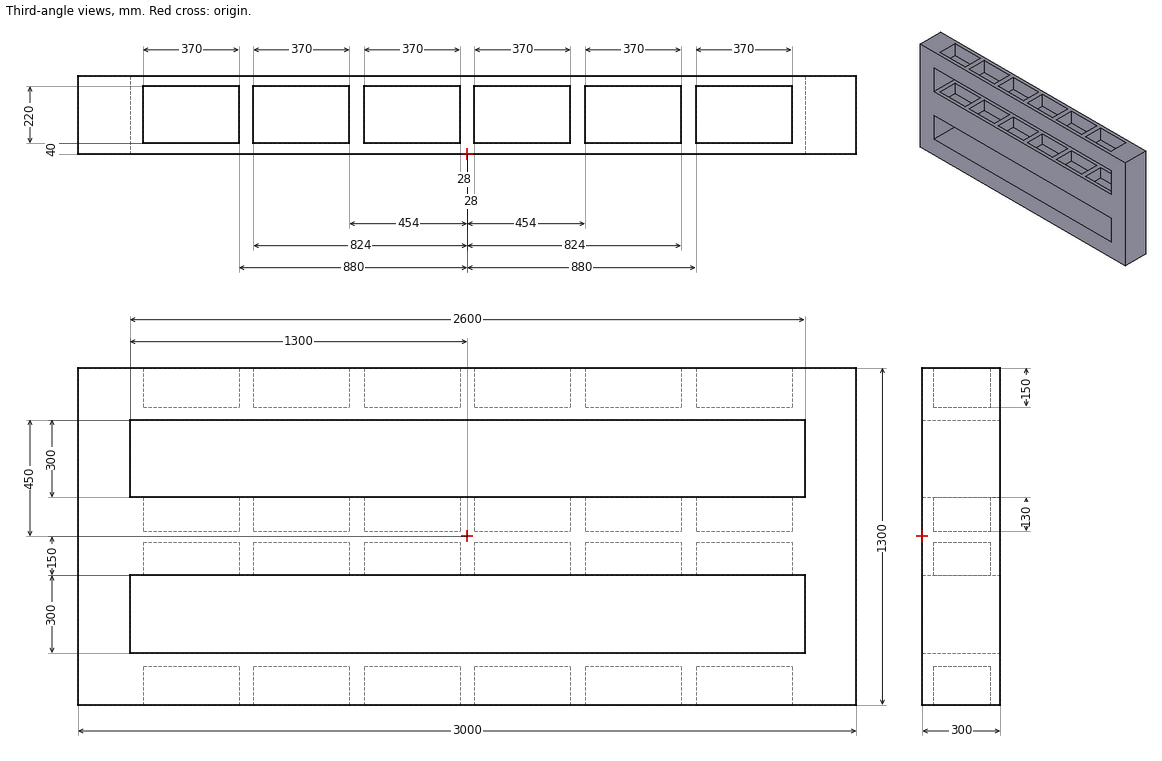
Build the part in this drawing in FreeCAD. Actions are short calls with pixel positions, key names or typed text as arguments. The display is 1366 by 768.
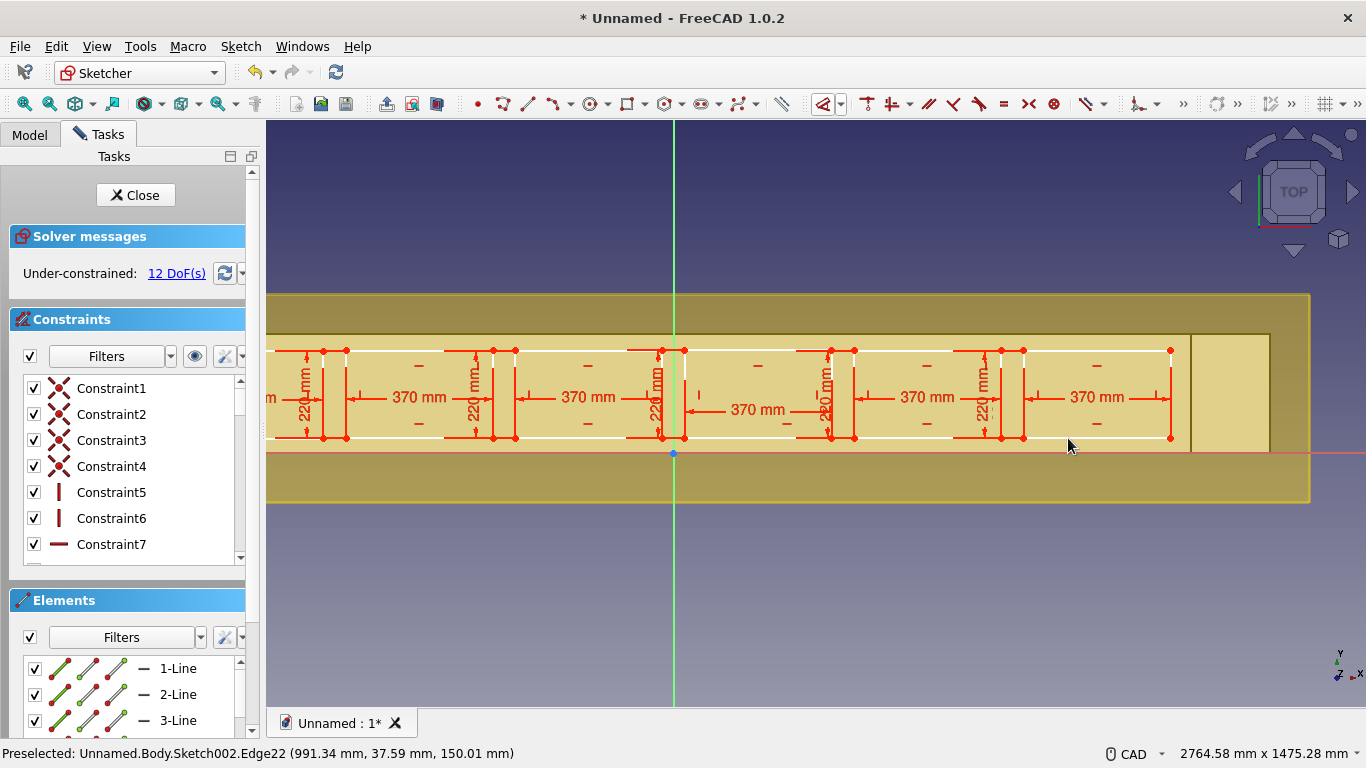
scroll(898, 438, down, 2)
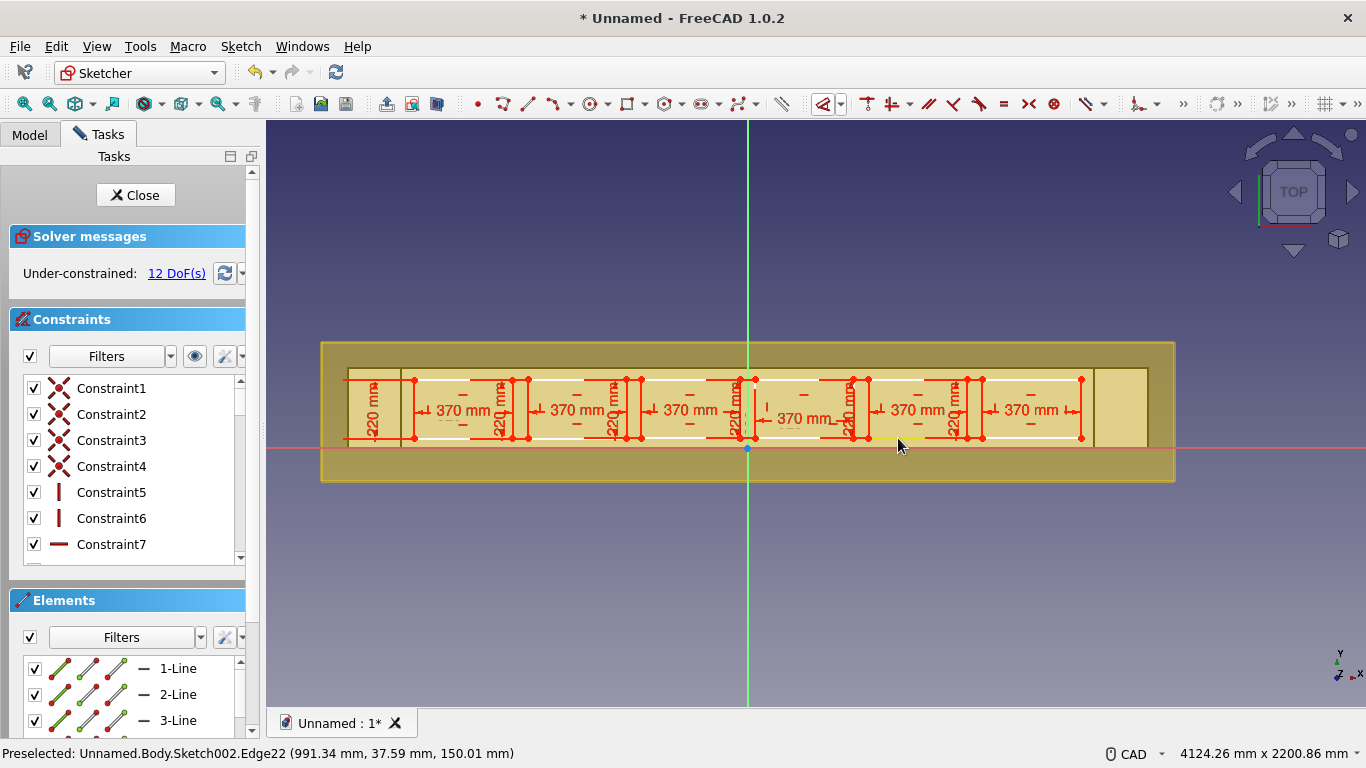
scroll(414, 439, up, 7)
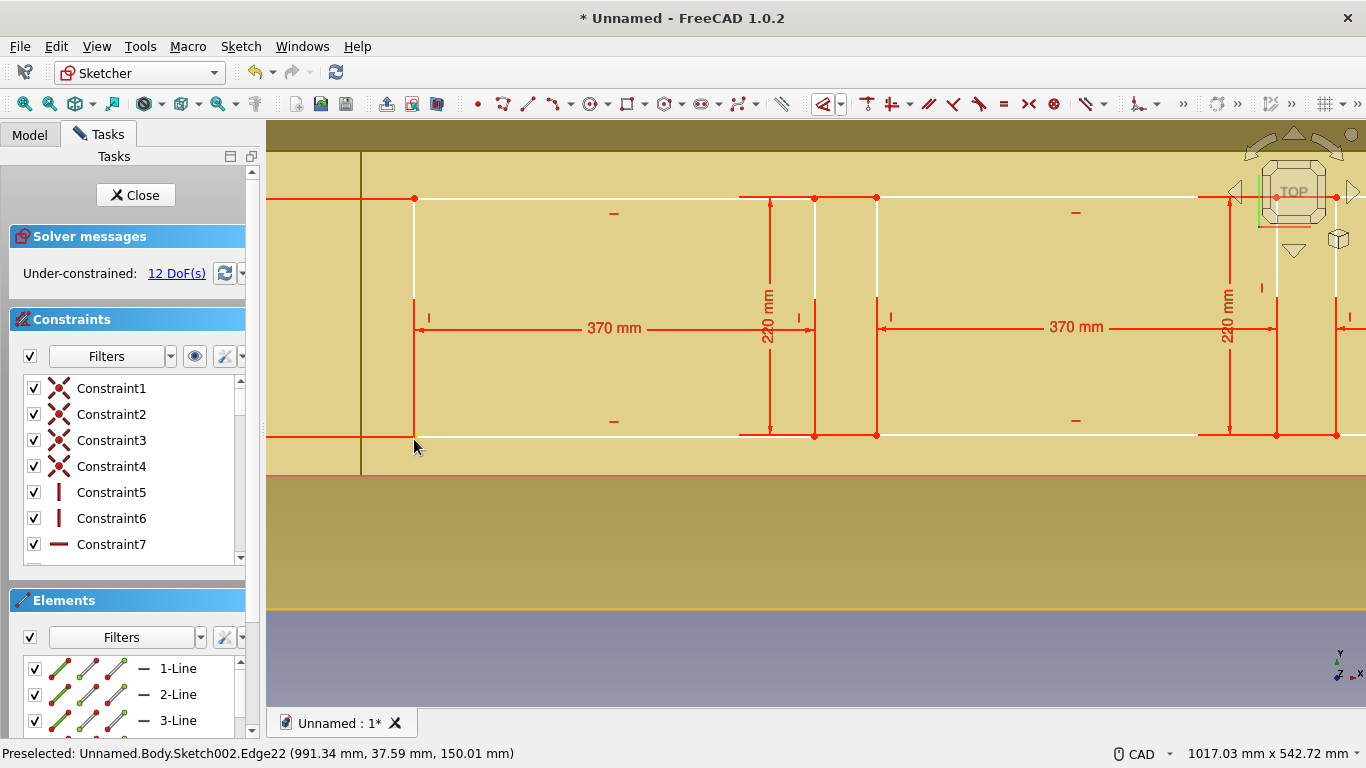
click(414, 437)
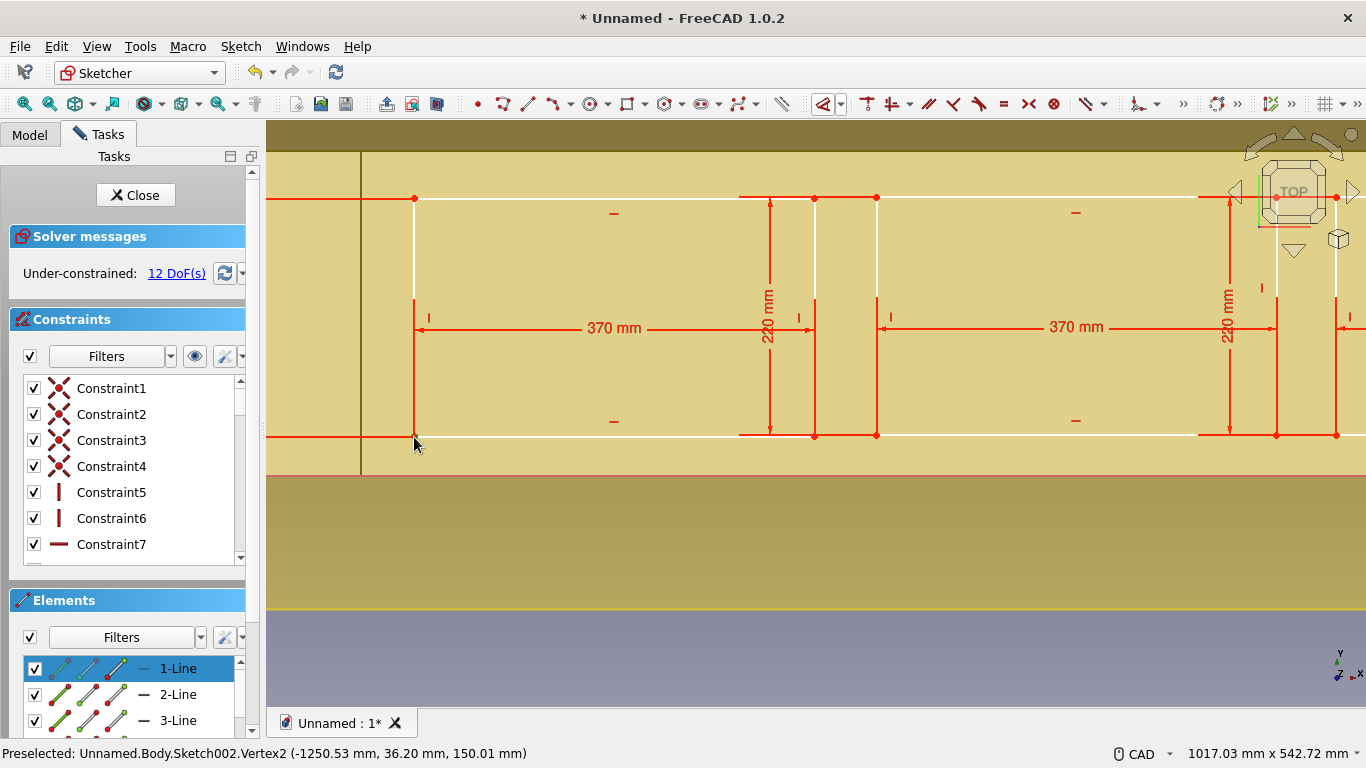
key(i)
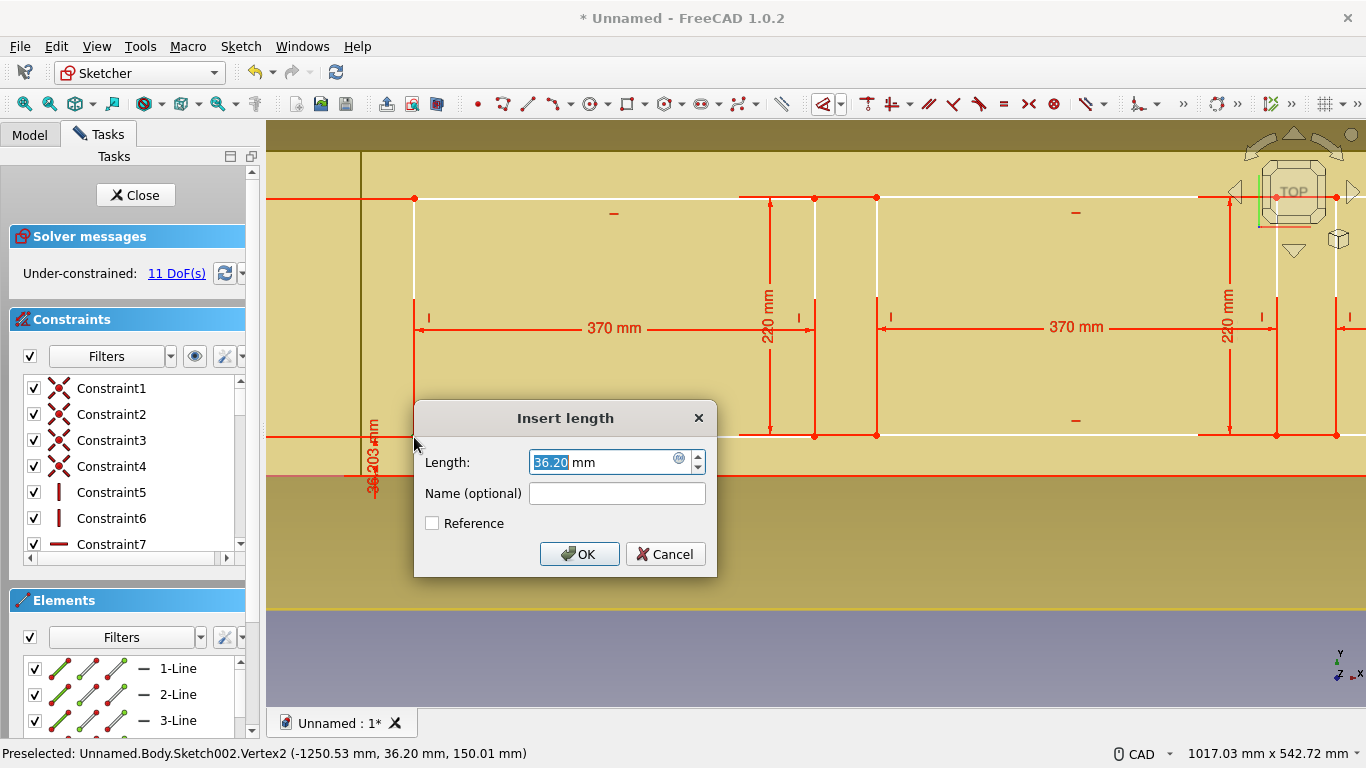
text(40)
key(Return)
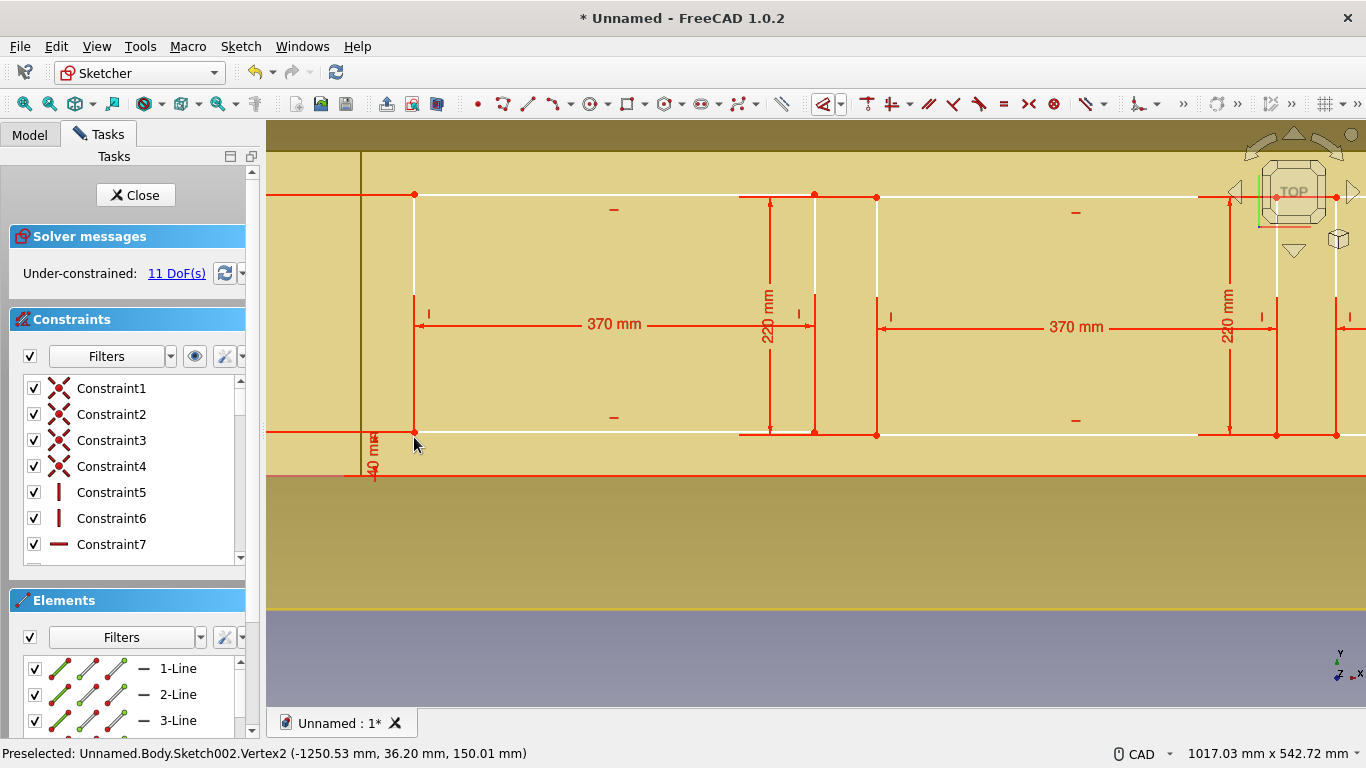
click(877, 435)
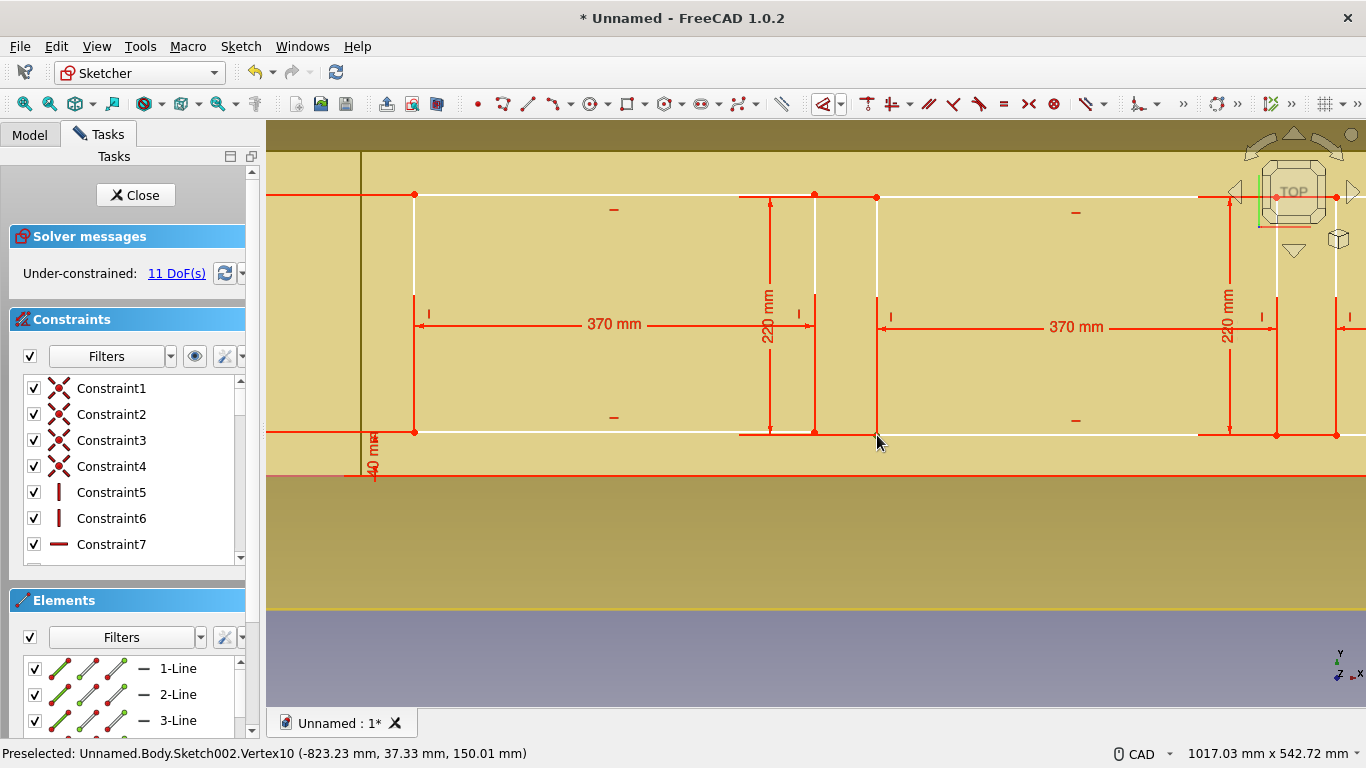
key(i)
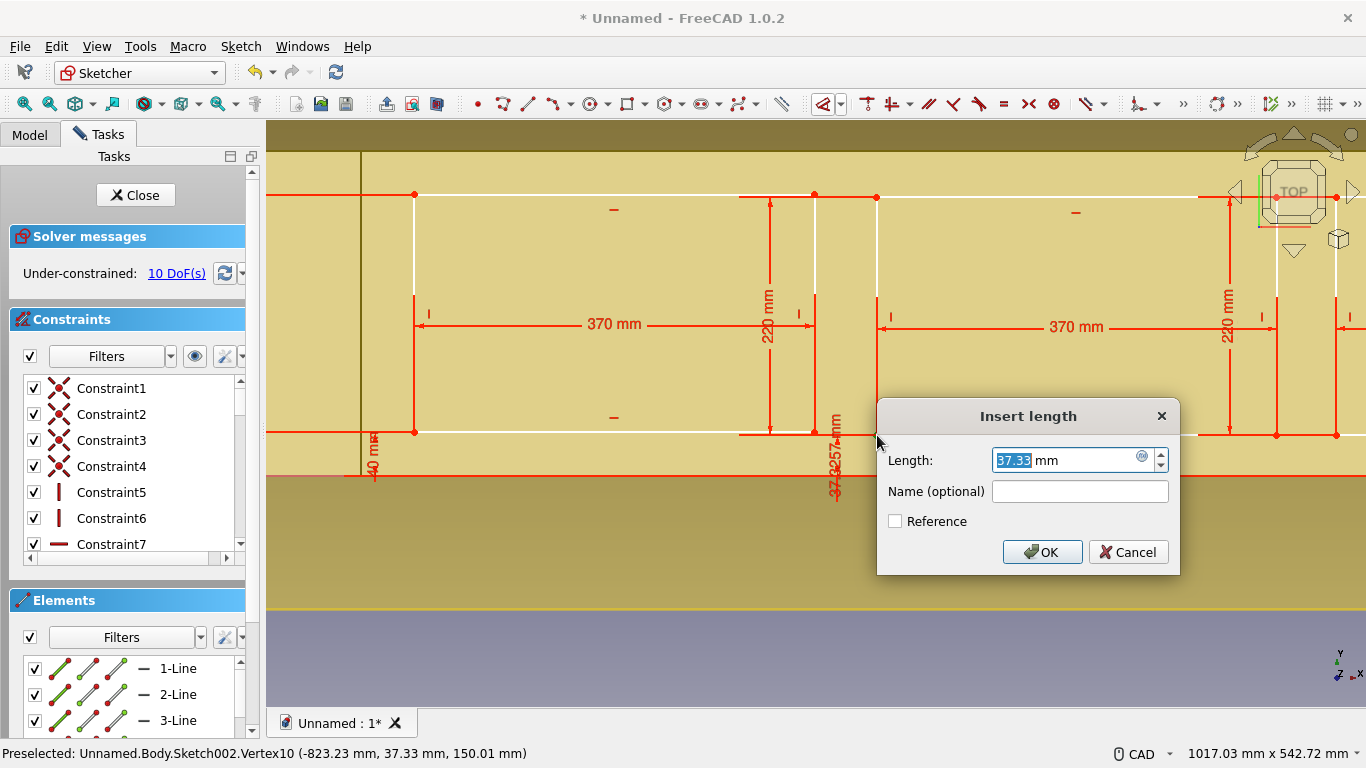
text(40)
key(Return)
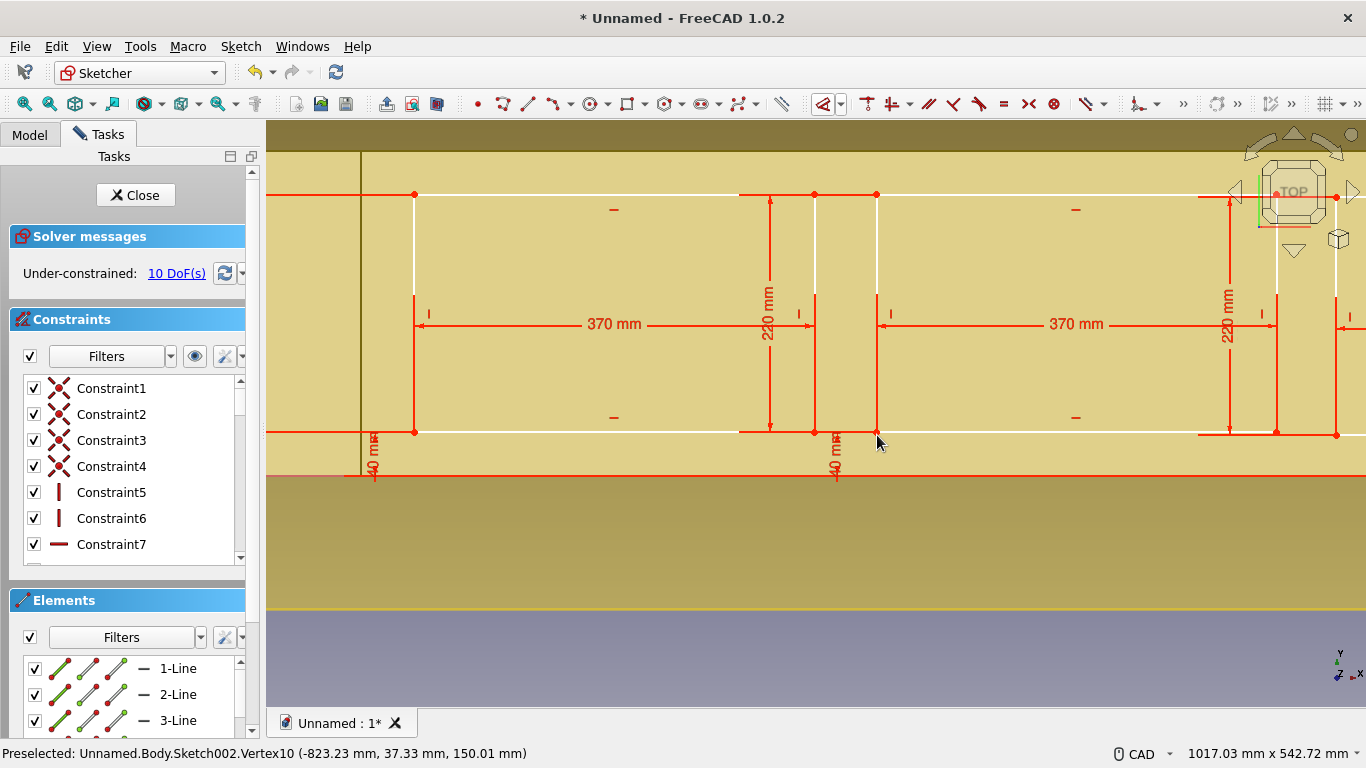
scroll(414, 439, down, 7)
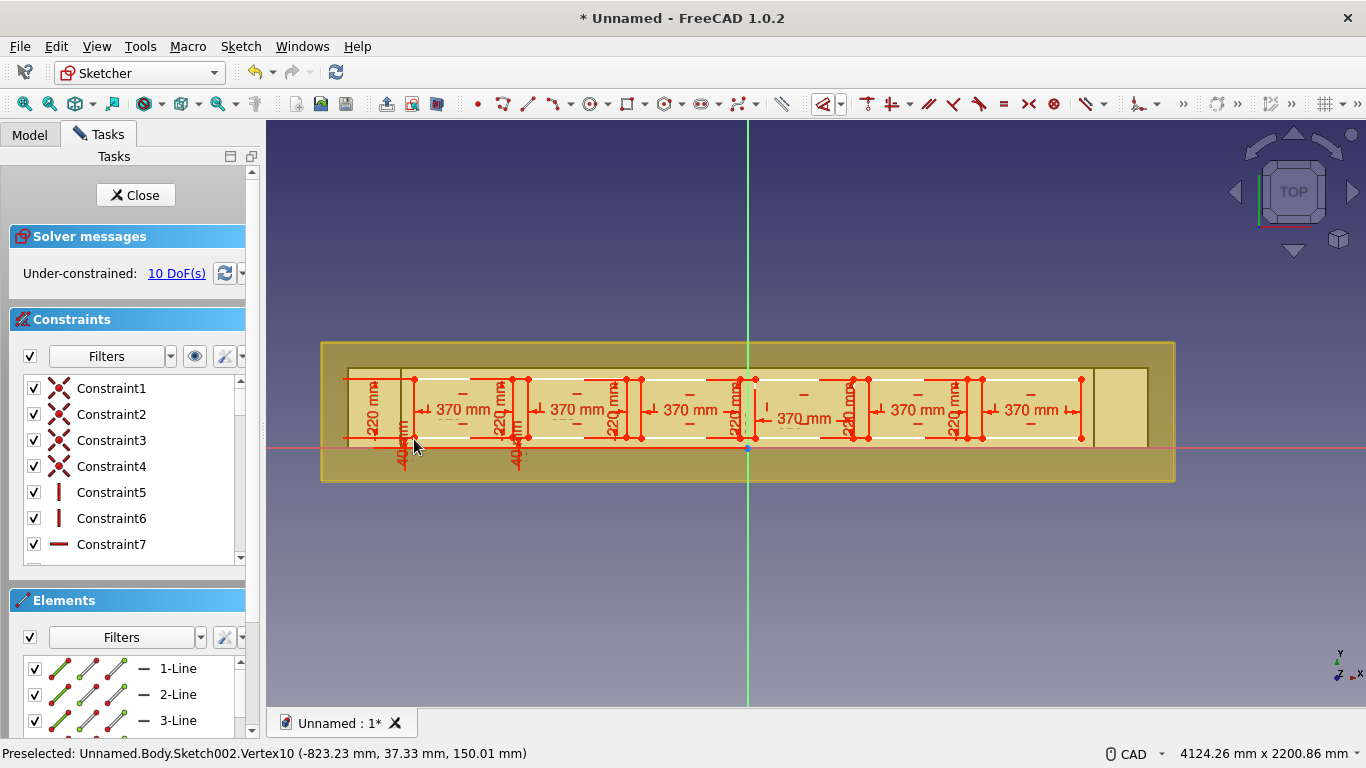
scroll(641, 438, up, 7)